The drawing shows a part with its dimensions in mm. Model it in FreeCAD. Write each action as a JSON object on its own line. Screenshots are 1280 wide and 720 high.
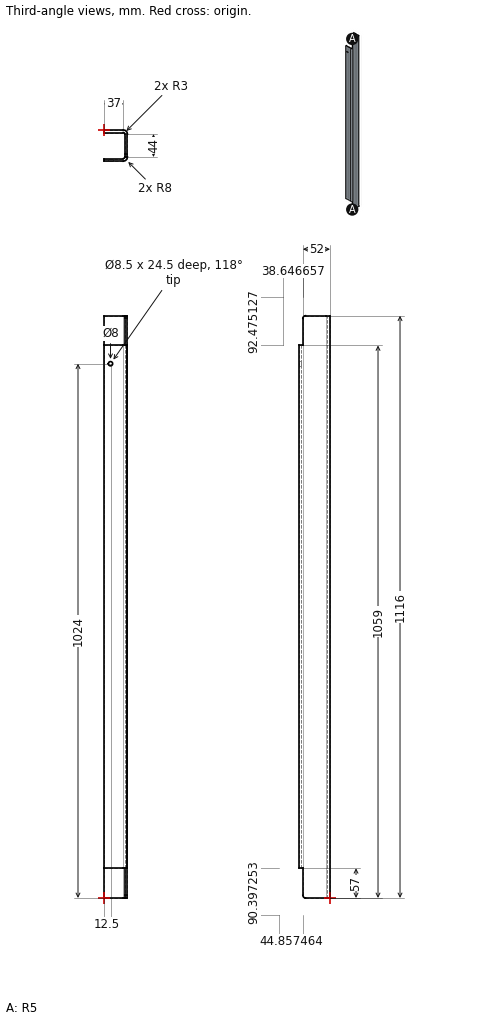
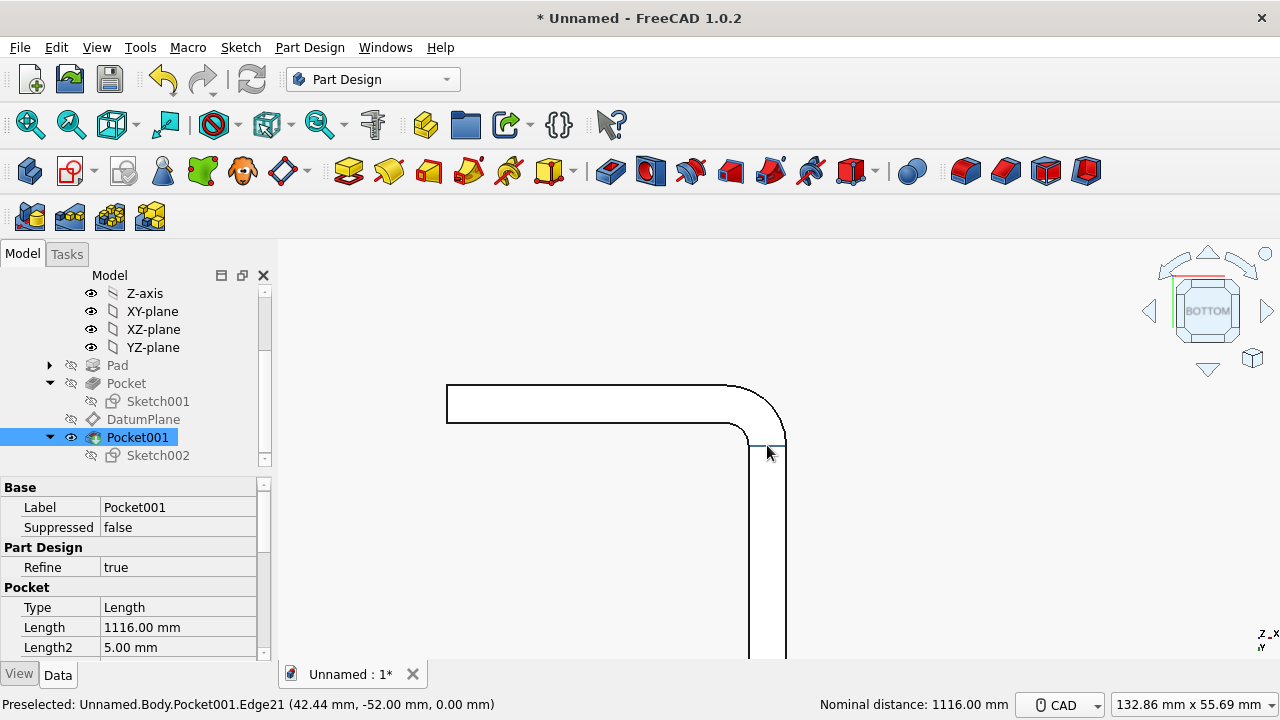
{"action": "left_click", "coordinate": [966, 172]}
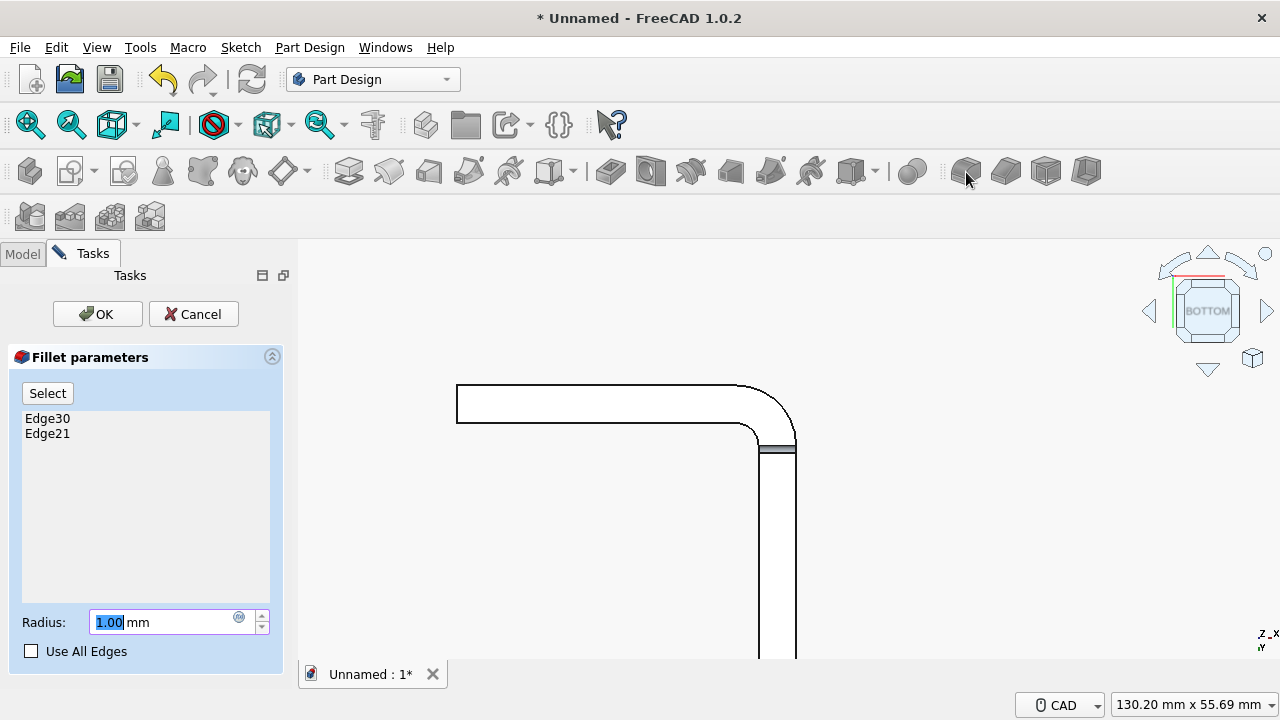
{"action": "type", "text": "5"}
{"action": "key", "text": "Tab"}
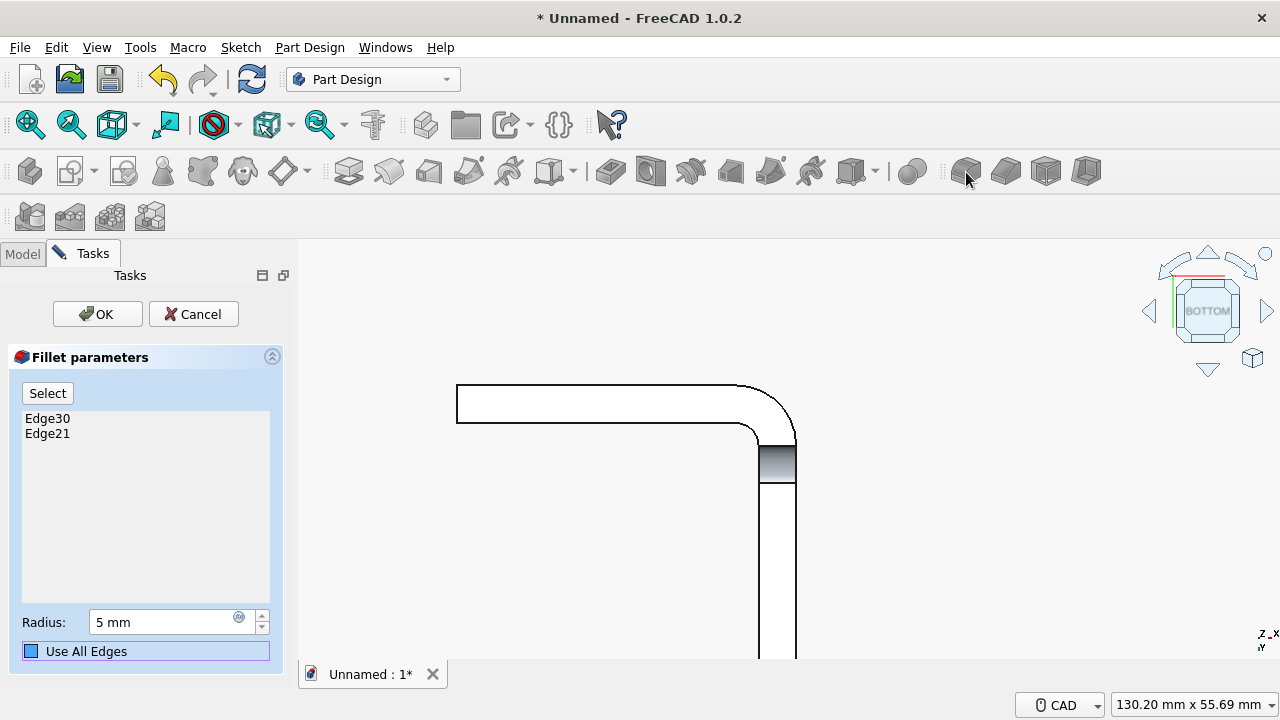
{"action": "left_click", "coordinate": [98, 314]}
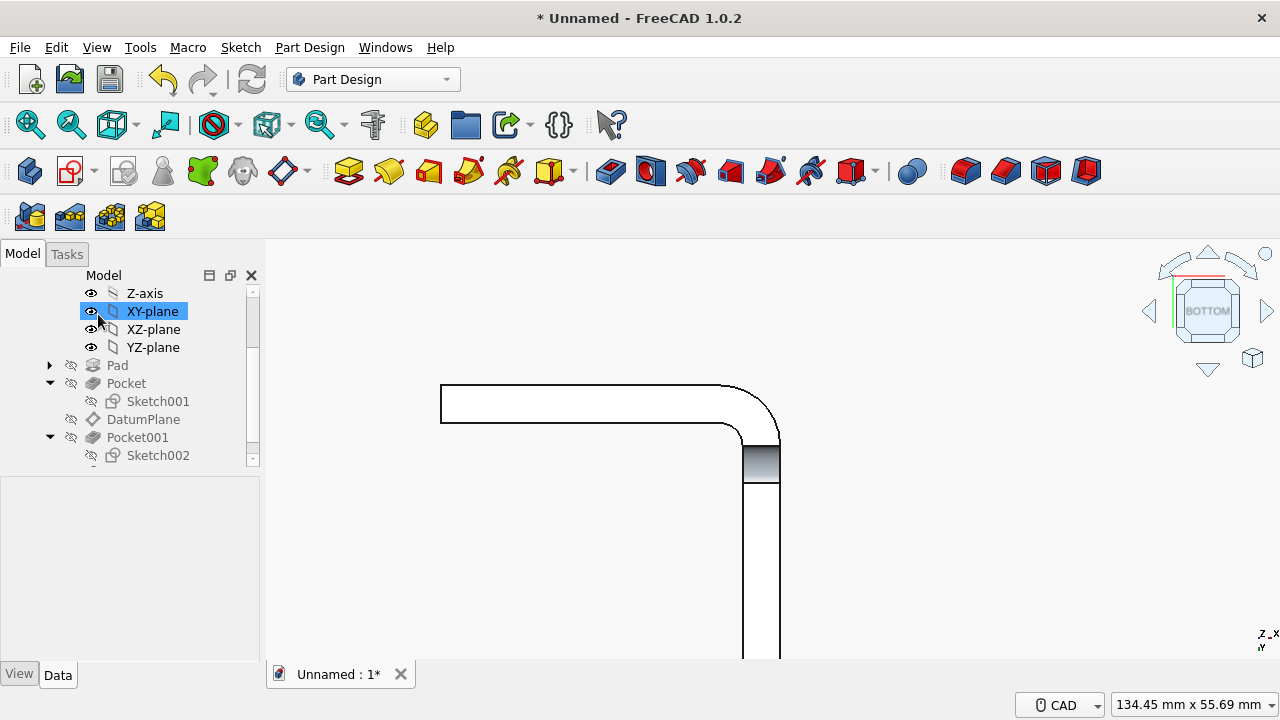
{"action": "left_click", "coordinate": [32, 126]}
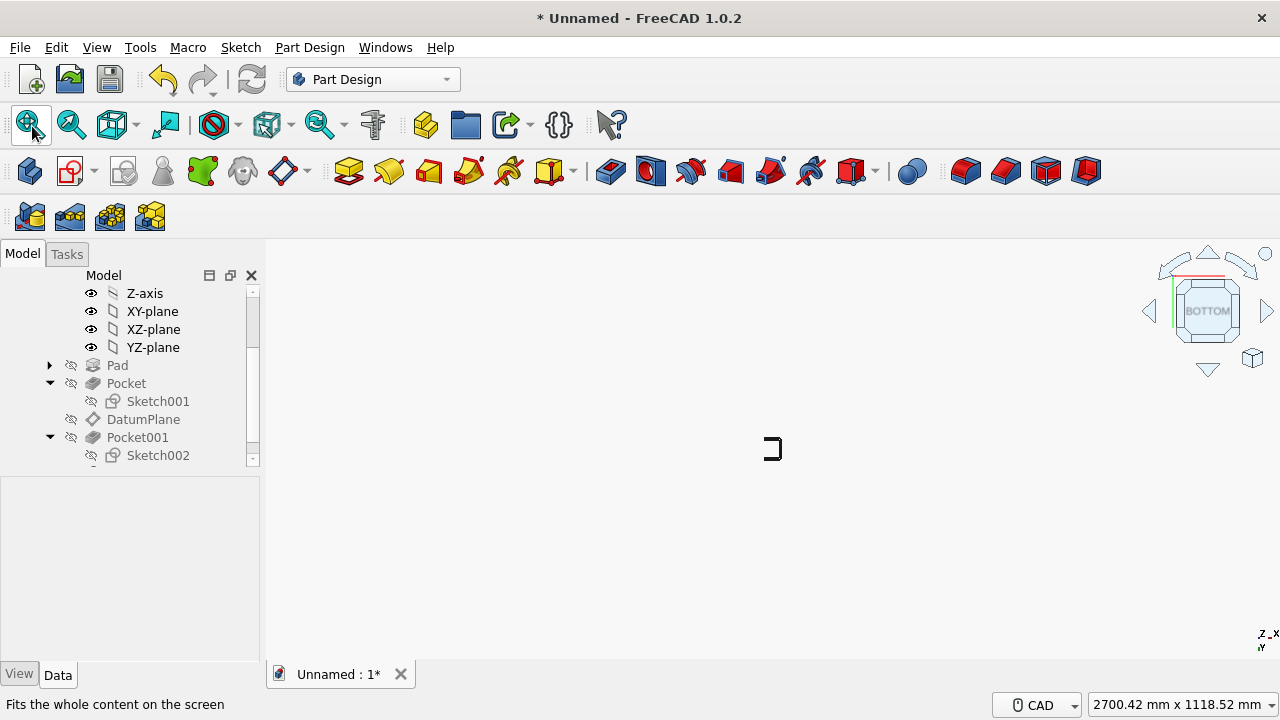
{"action": "scroll", "coordinate": [160, 379], "scroll_direction": "down", "scroll_amount": 3}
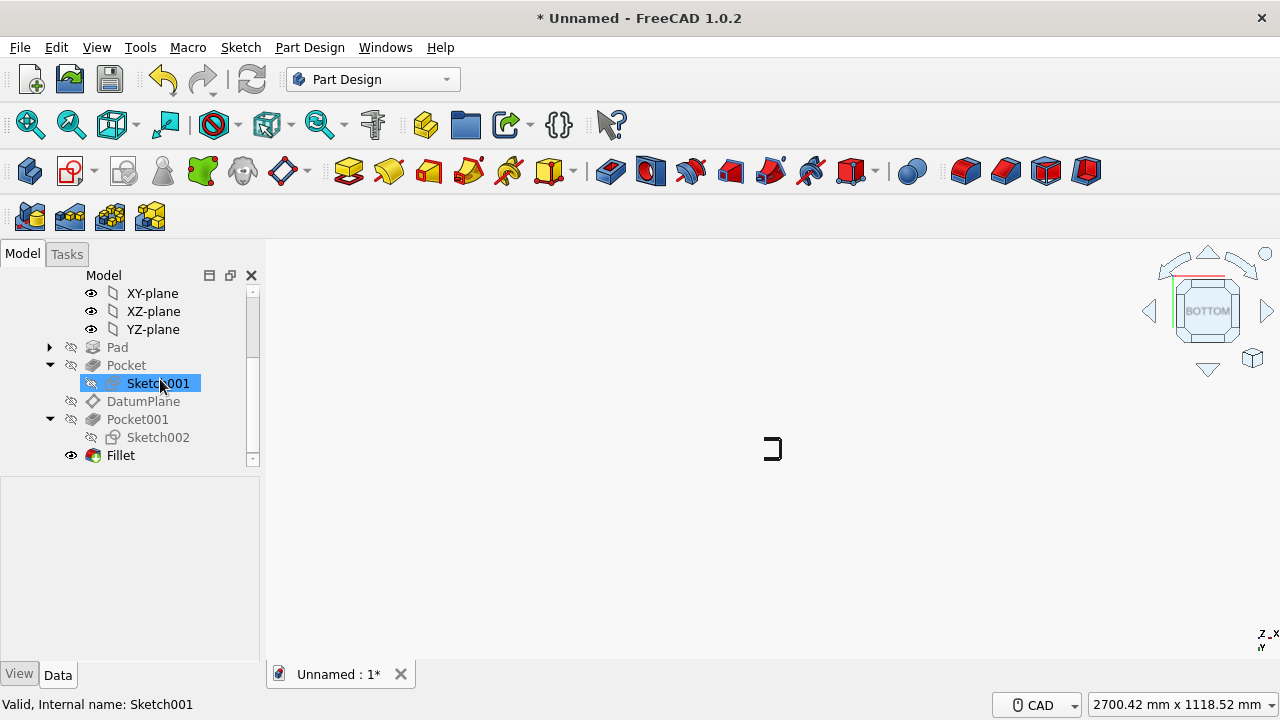
{"action": "scroll", "coordinate": [160, 379], "scroll_direction": "up", "scroll_amount": 15}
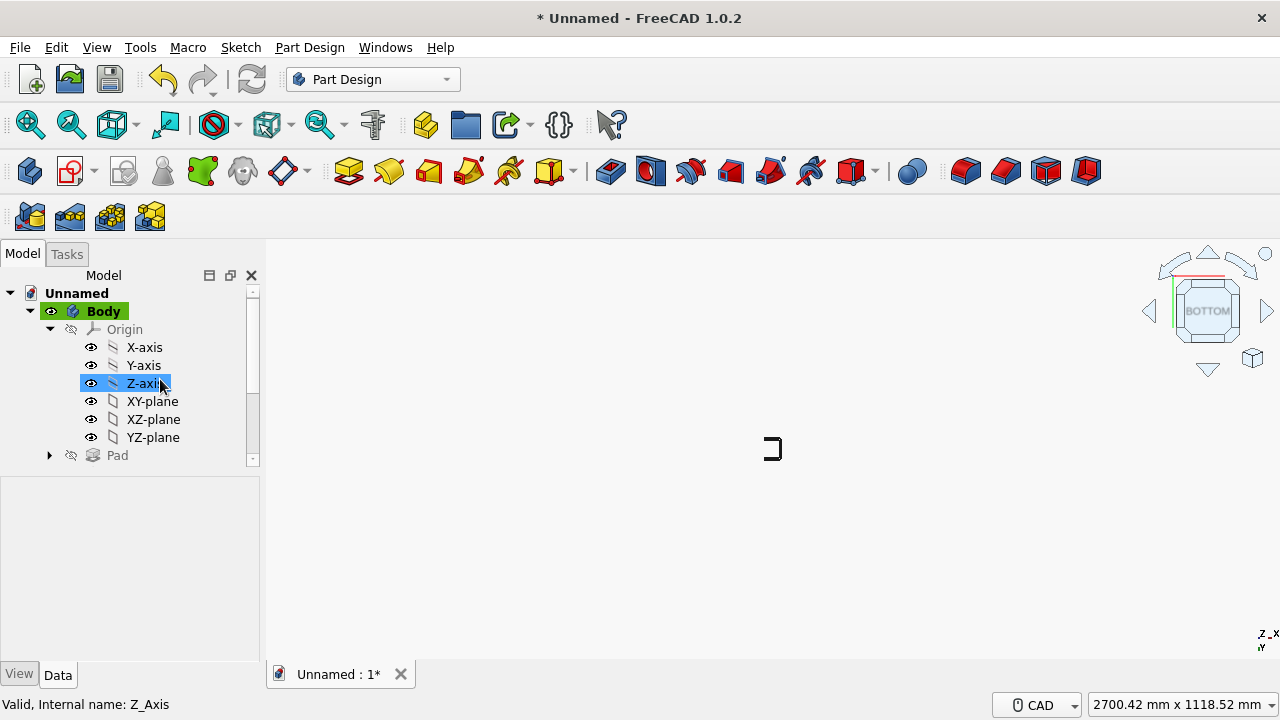
{"action": "left_click", "coordinate": [136, 419]}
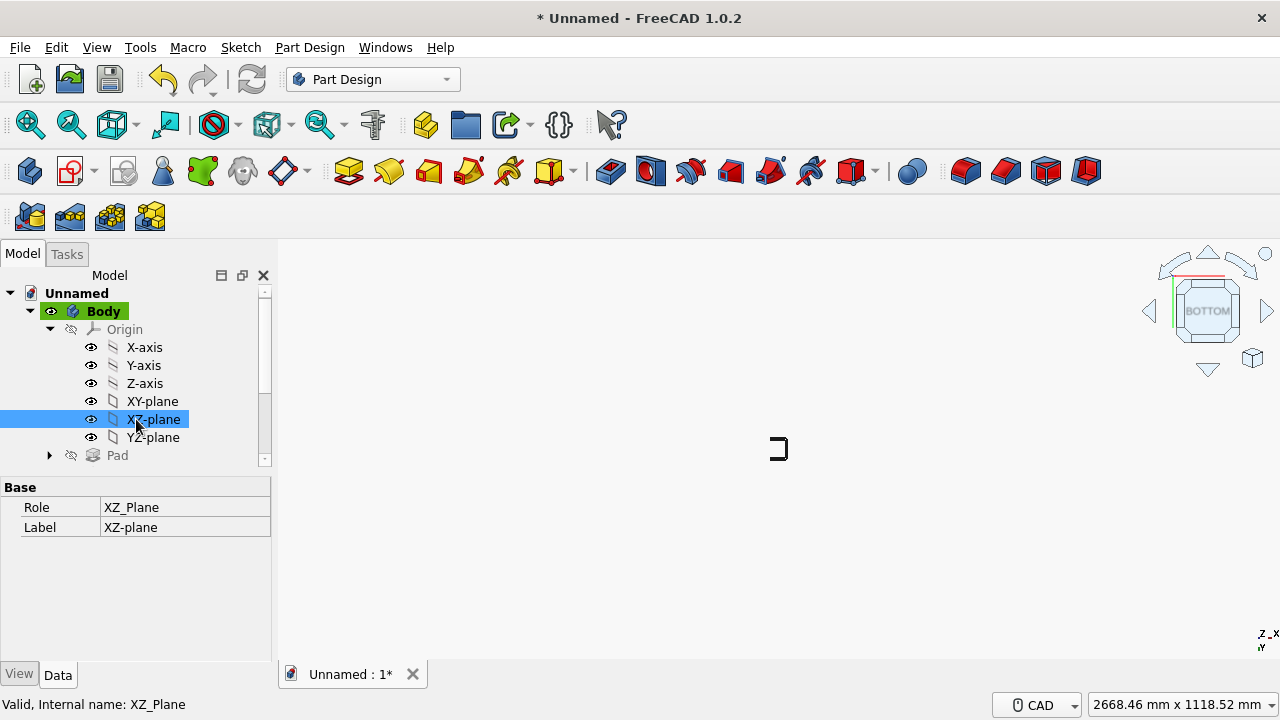
{"action": "left_click", "coordinate": [284, 172]}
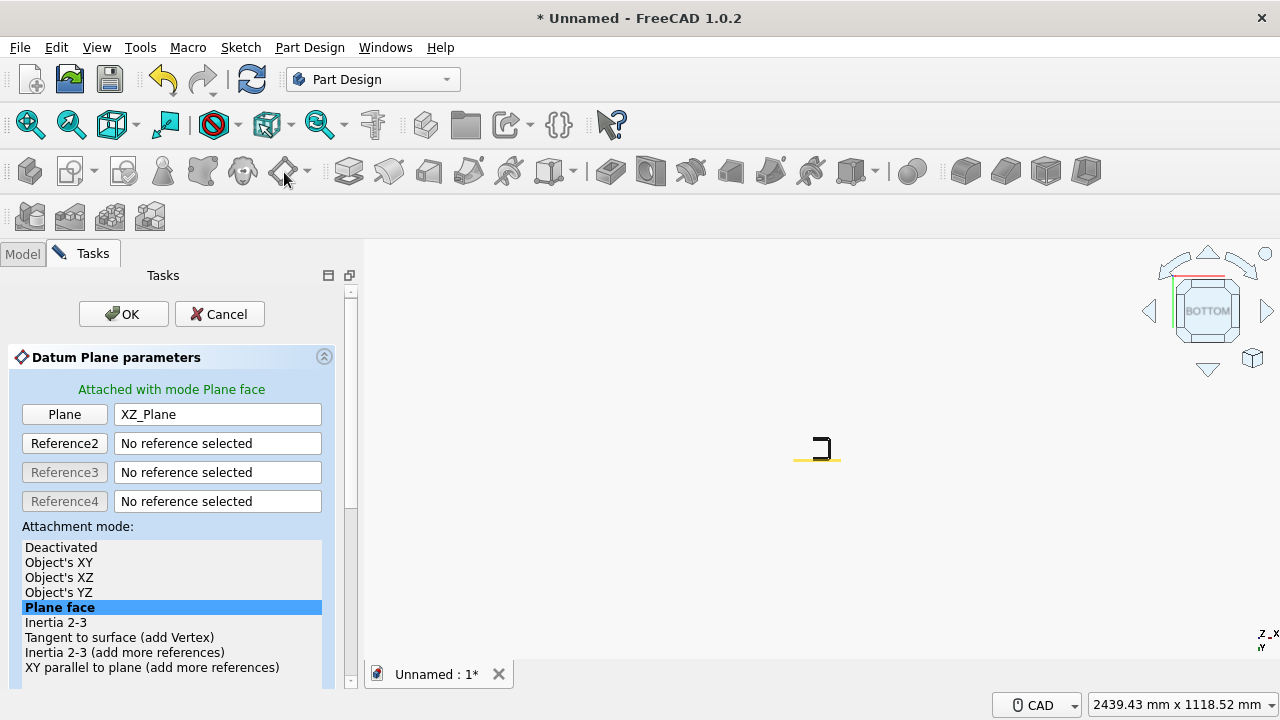
{"action": "scroll", "coordinate": [351, 486], "scroll_direction": "down", "scroll_amount": 4}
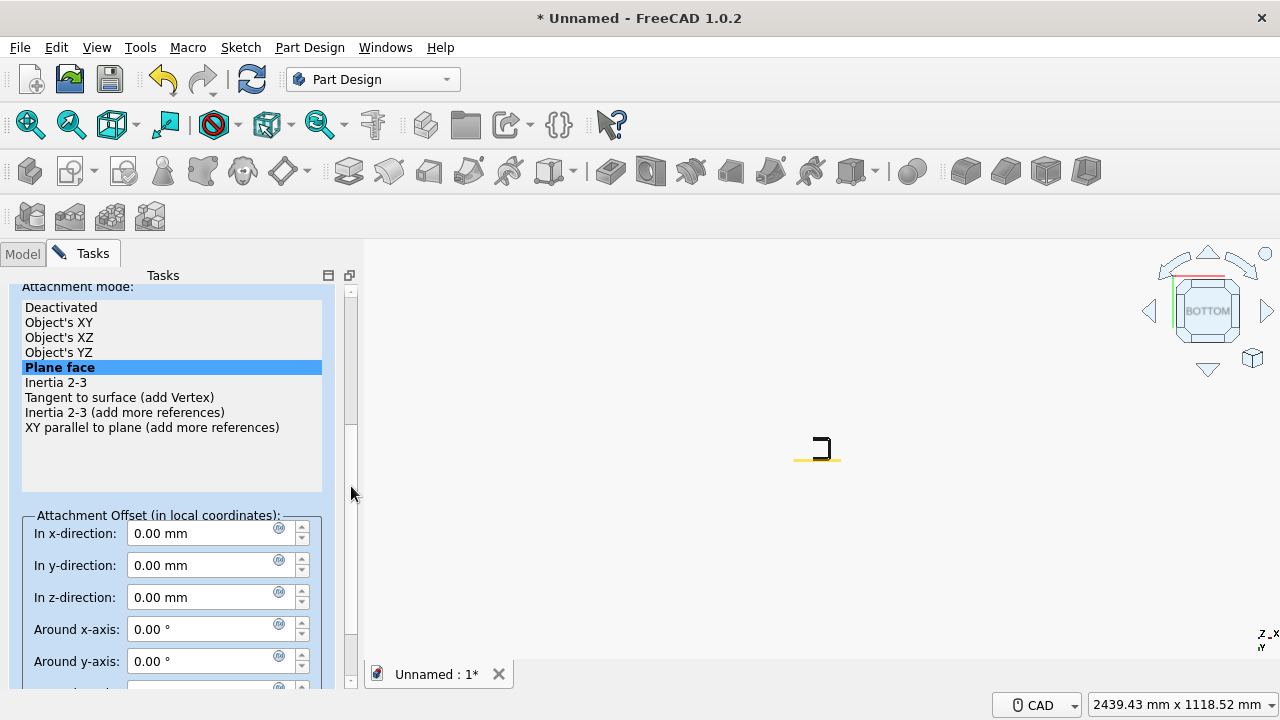
{"action": "triple_click", "coordinate": [210, 597]}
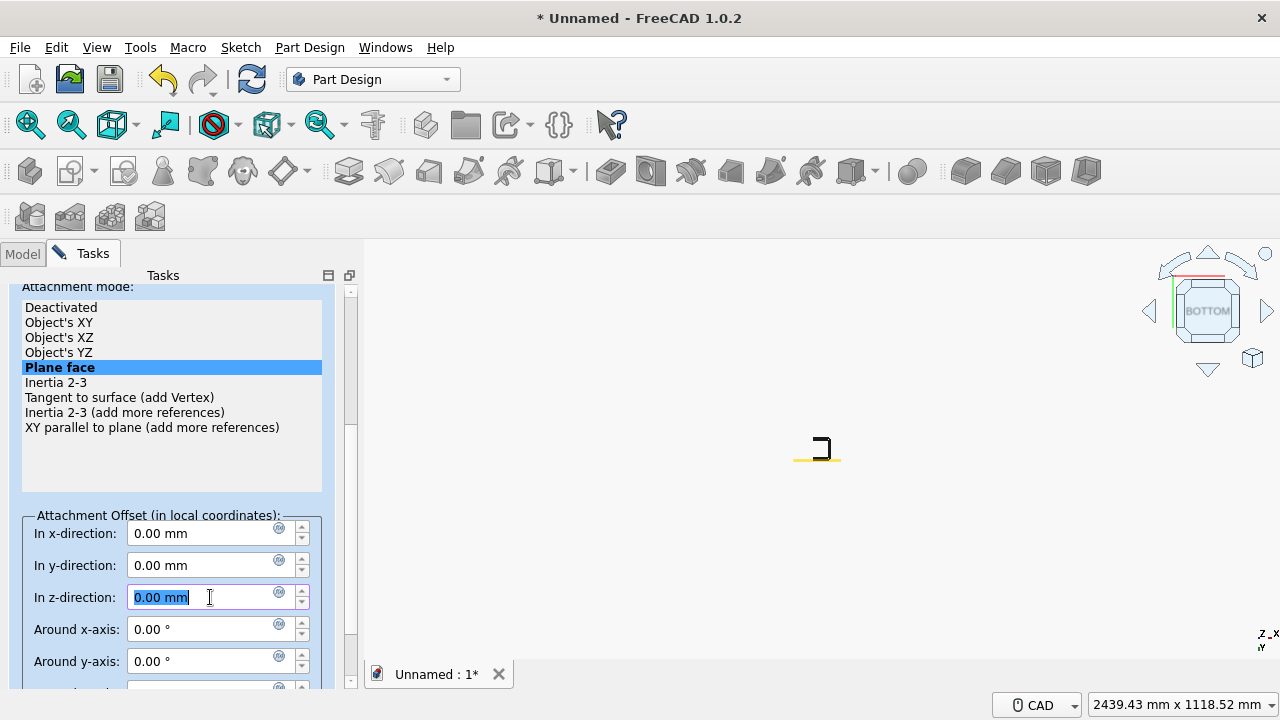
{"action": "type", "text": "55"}
{"action": "key", "text": "Tab"}